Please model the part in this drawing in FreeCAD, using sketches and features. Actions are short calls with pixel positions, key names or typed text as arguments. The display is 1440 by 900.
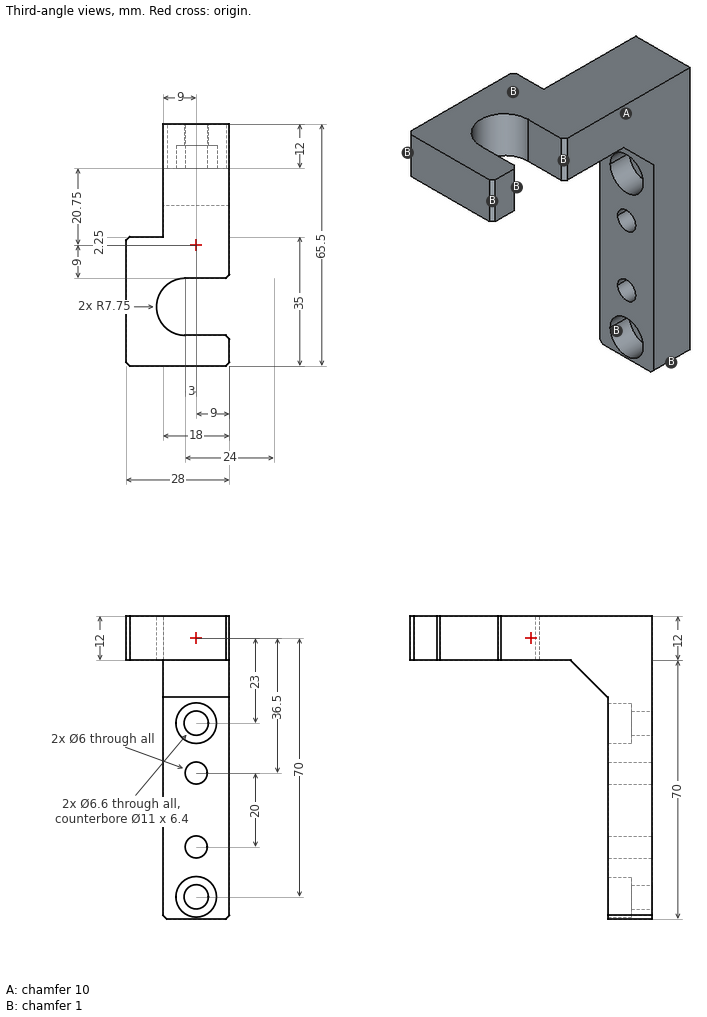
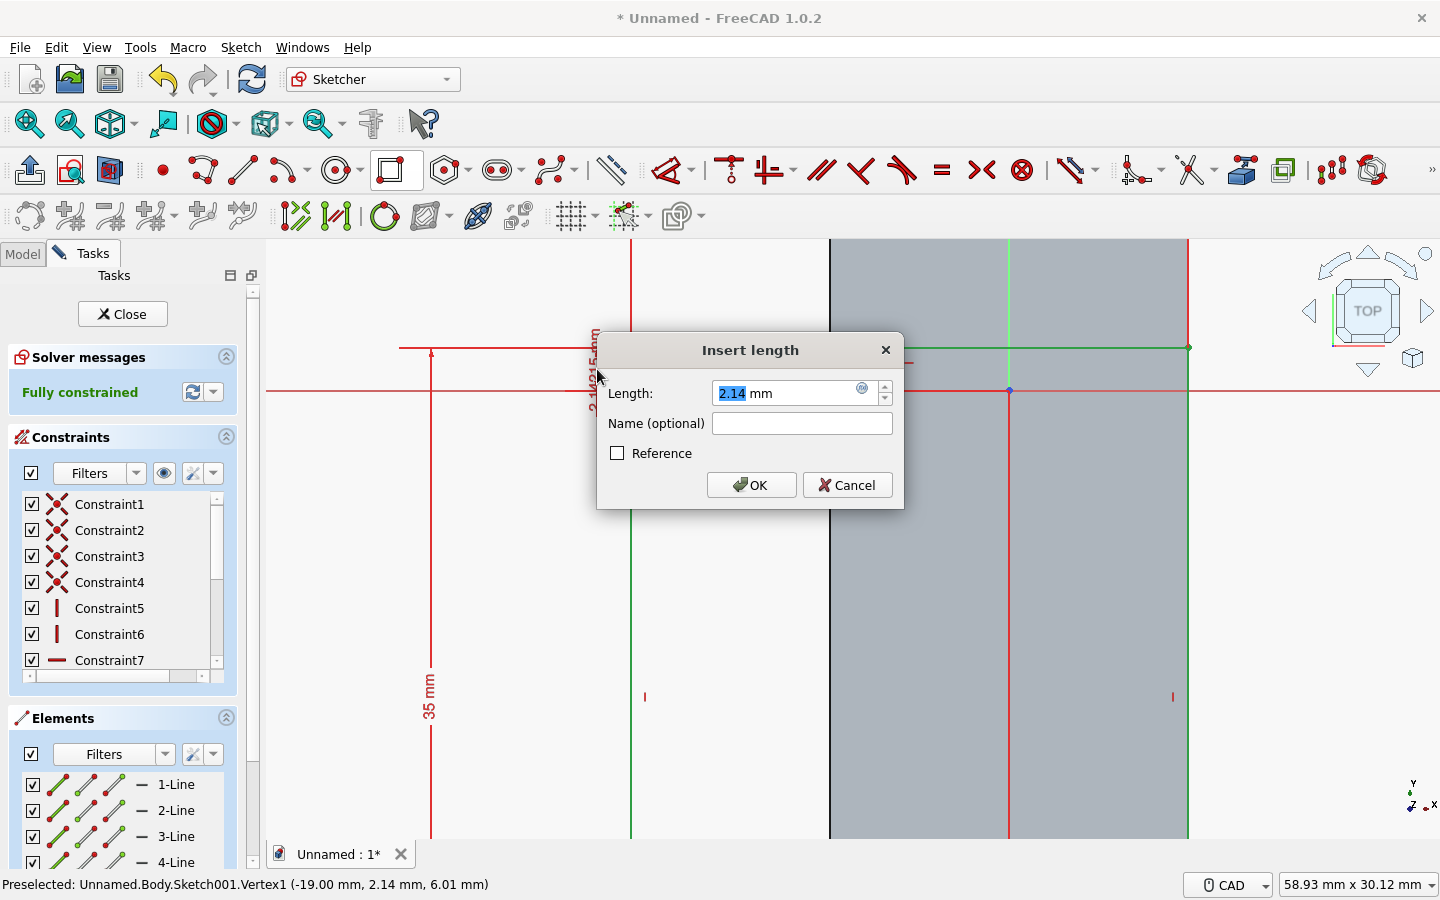
text(2.25)
key(Return)
key(Escape)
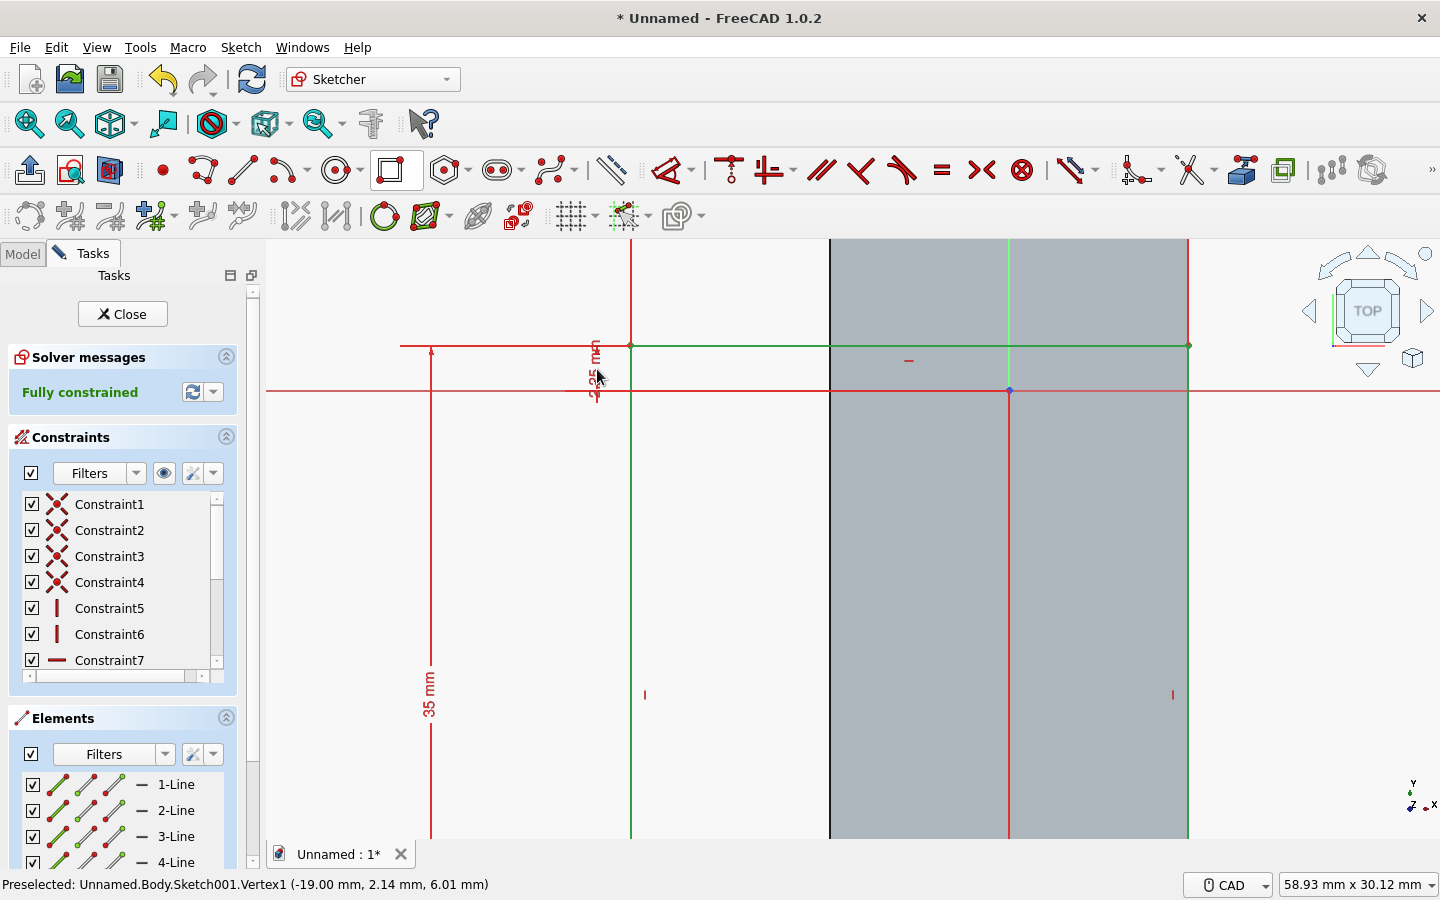
click(123, 314)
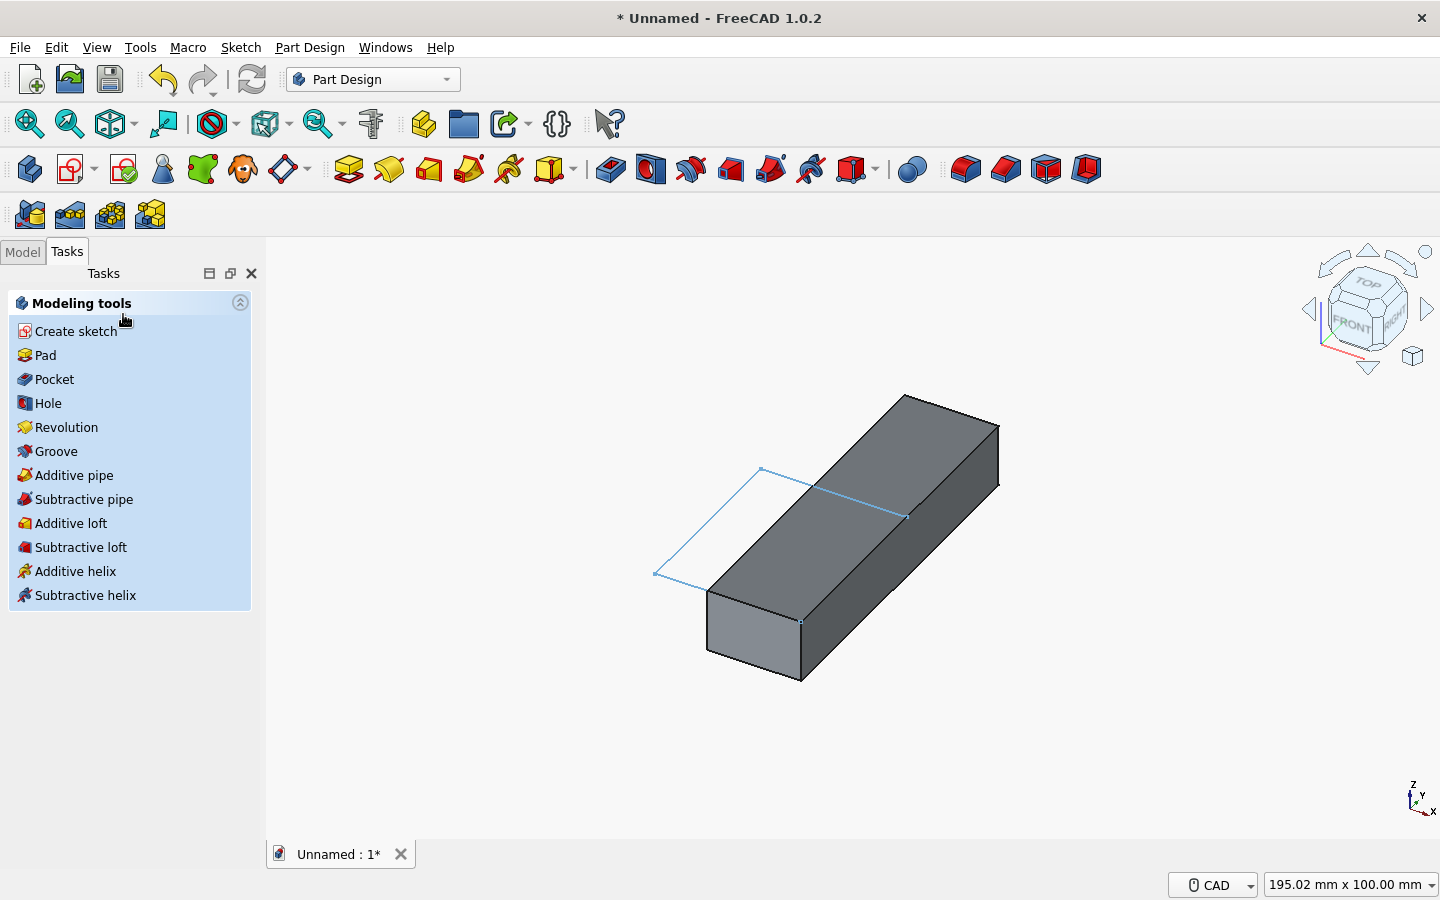
click(350, 170)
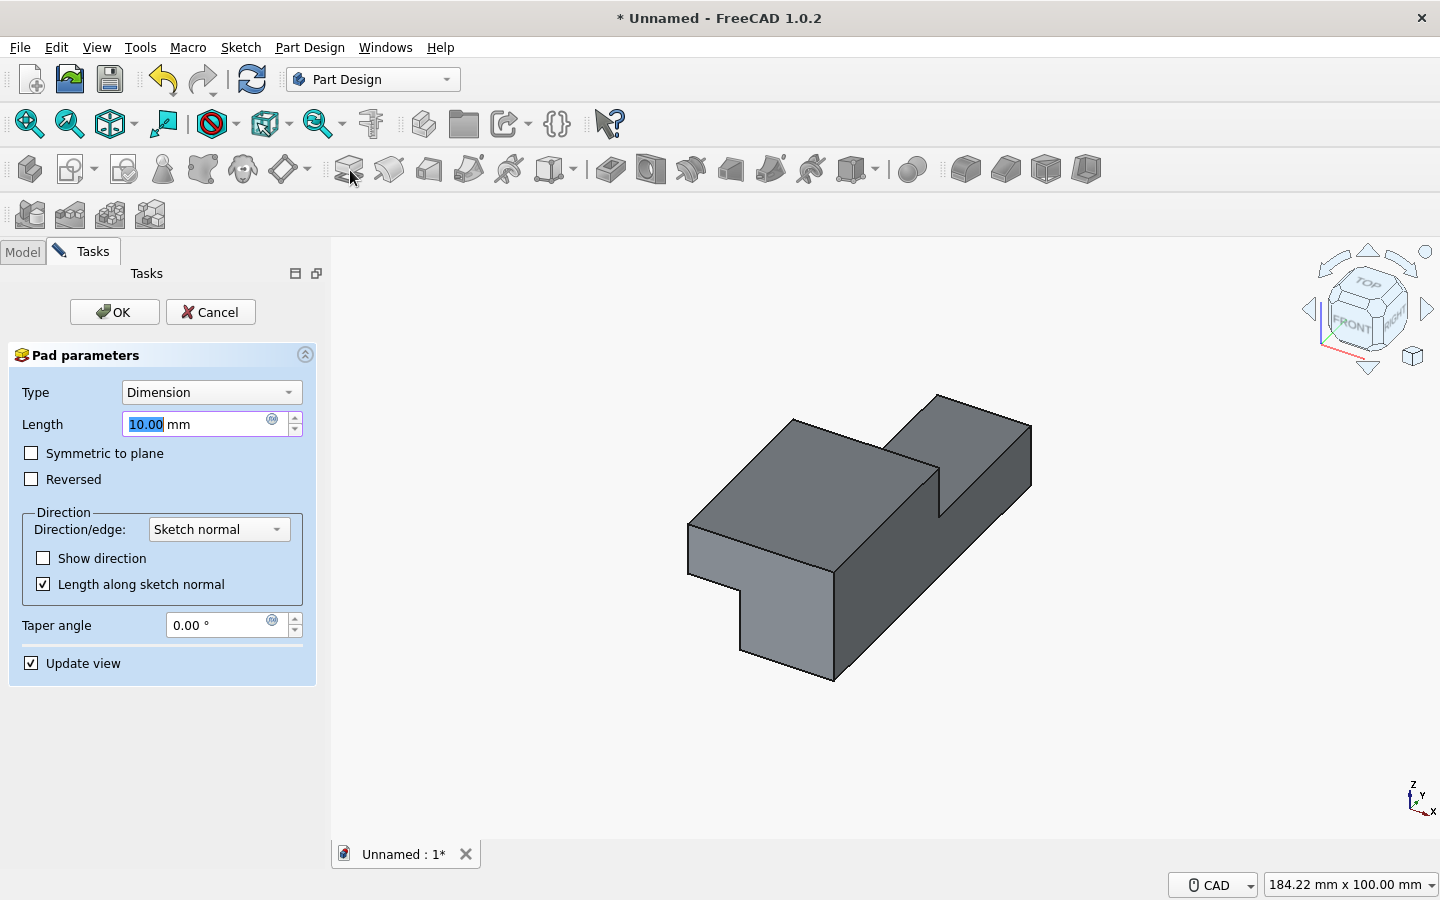
text(12)
key(Tab)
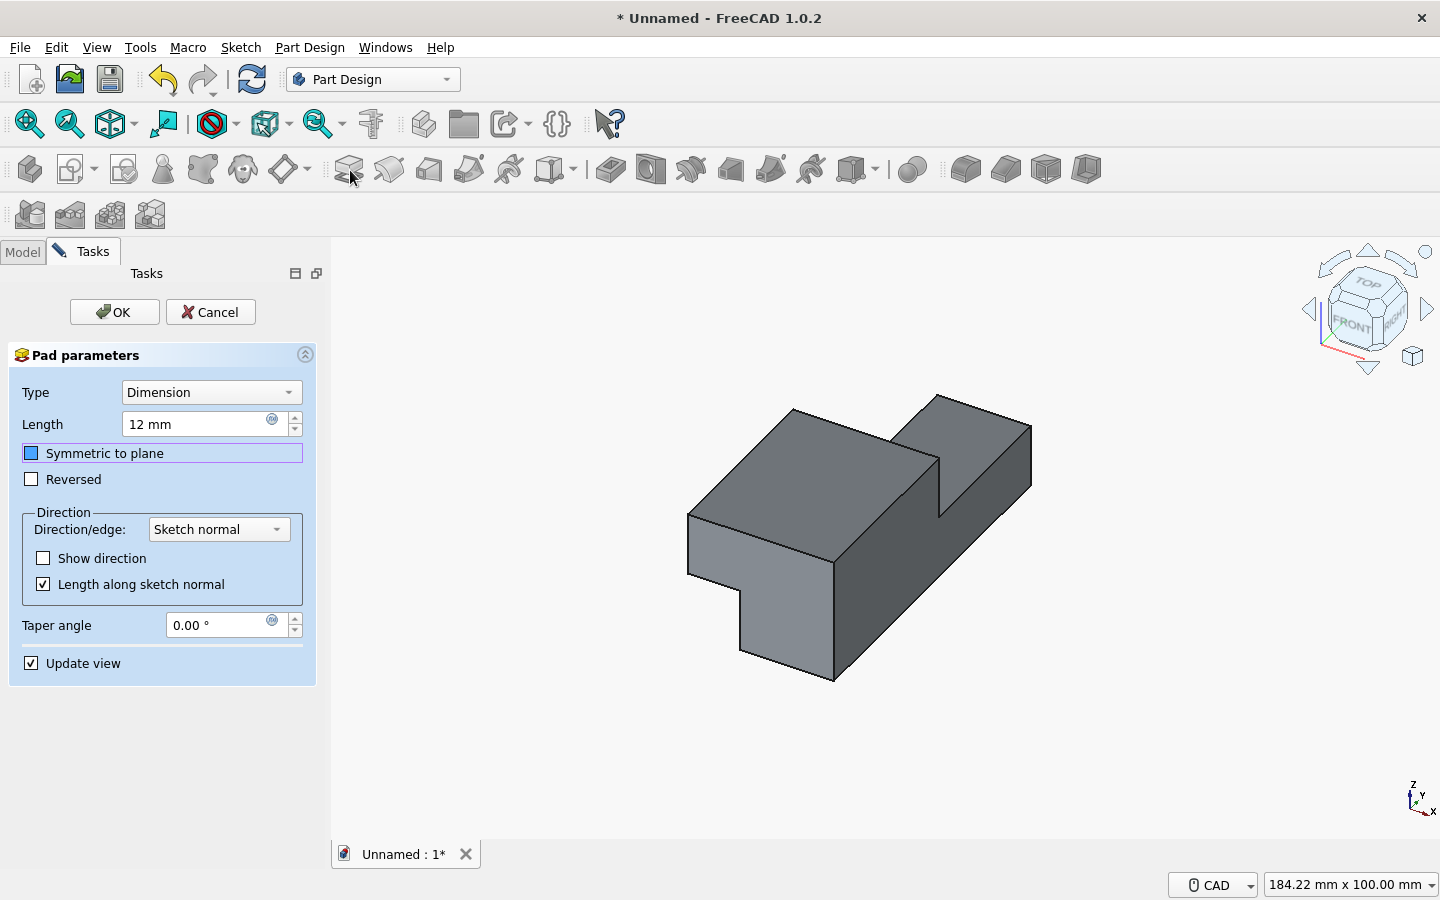
click(30, 479)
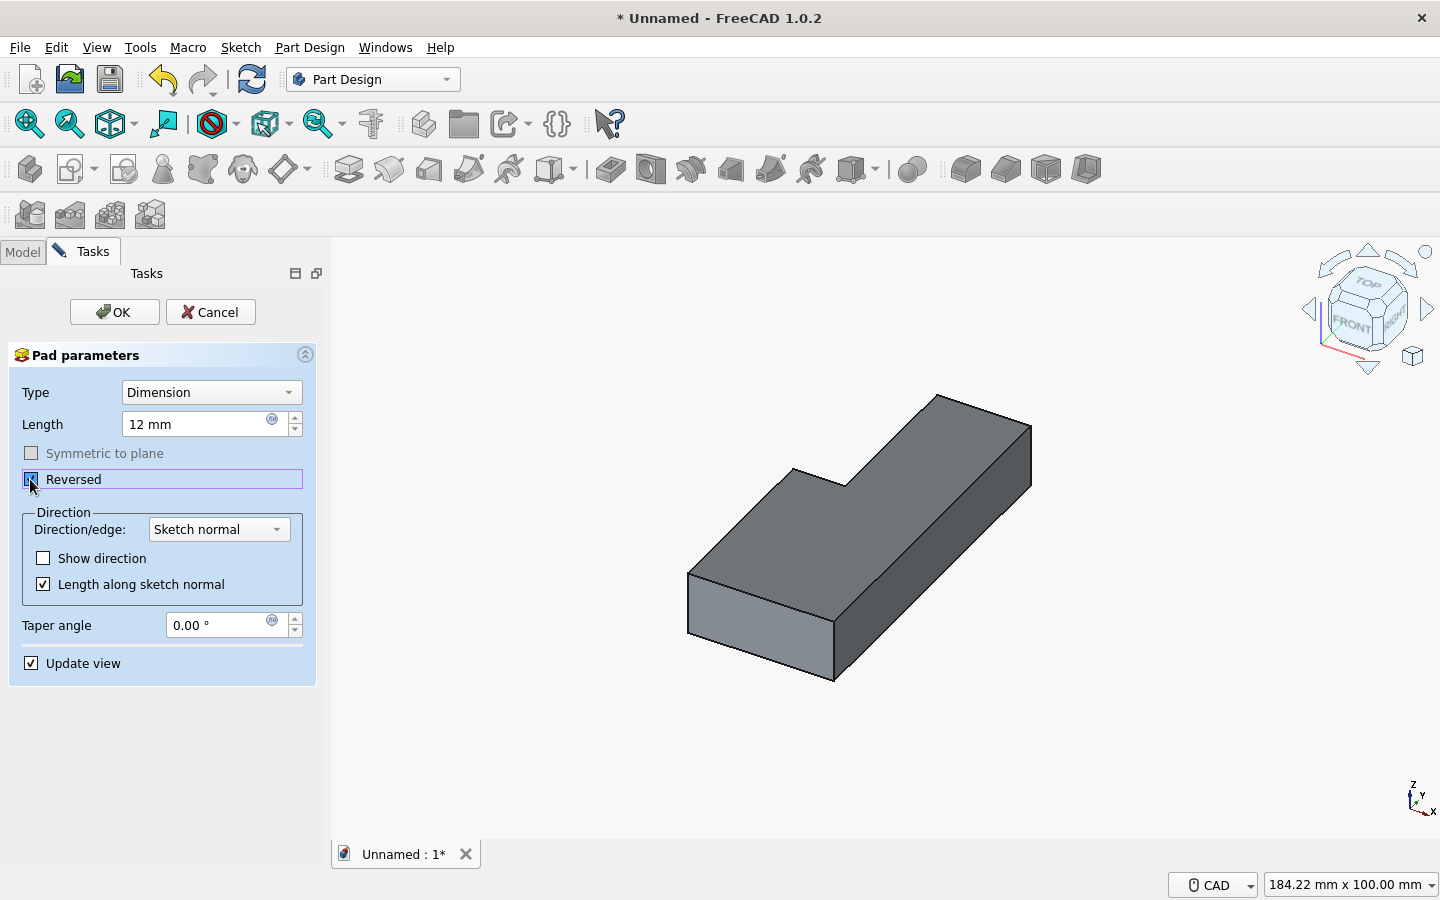
click(115, 312)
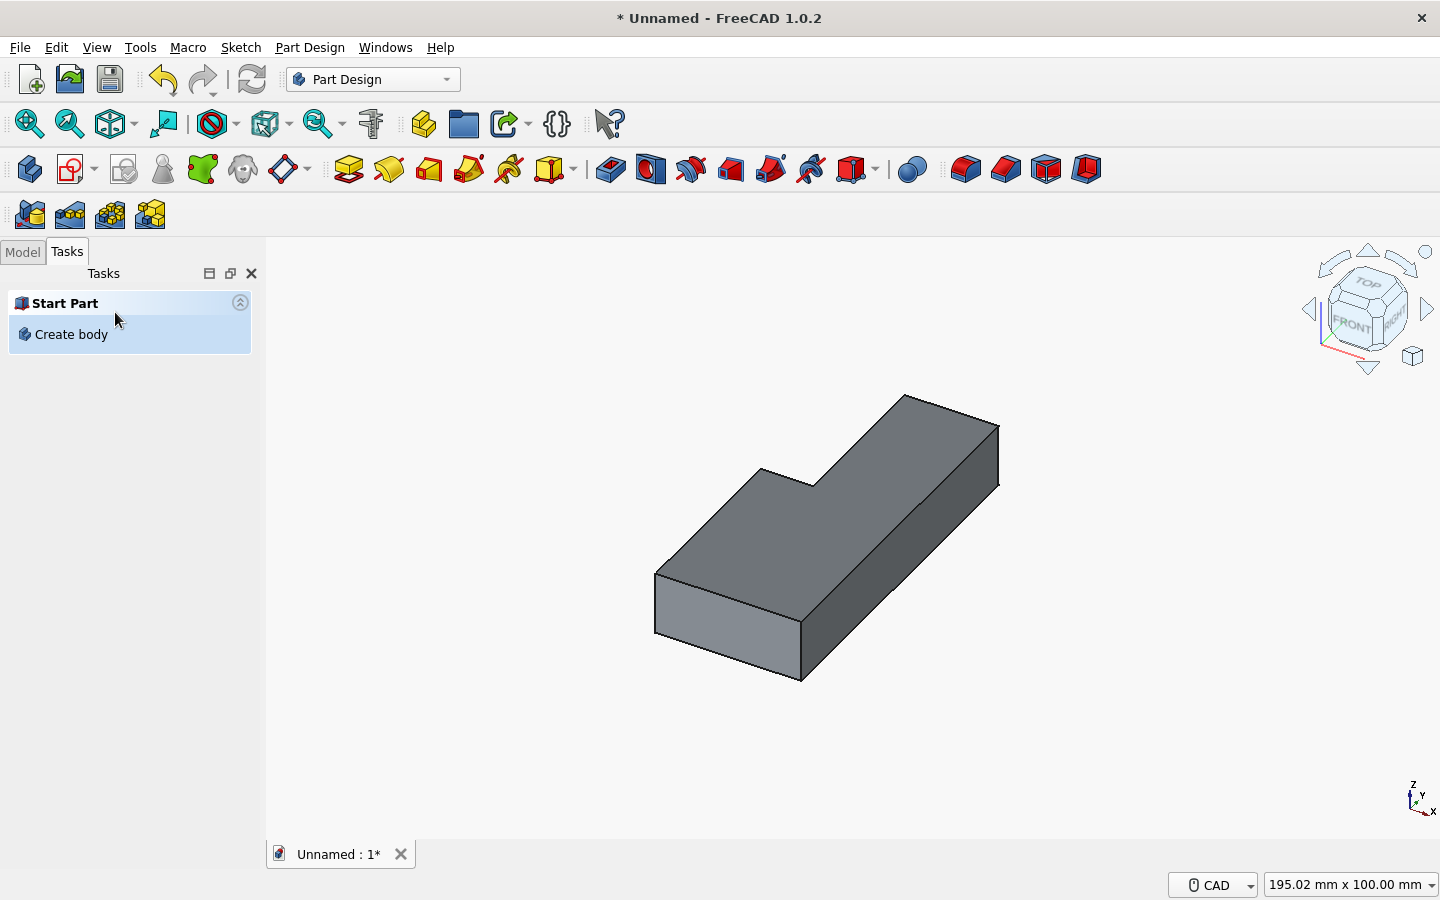
click(771, 555)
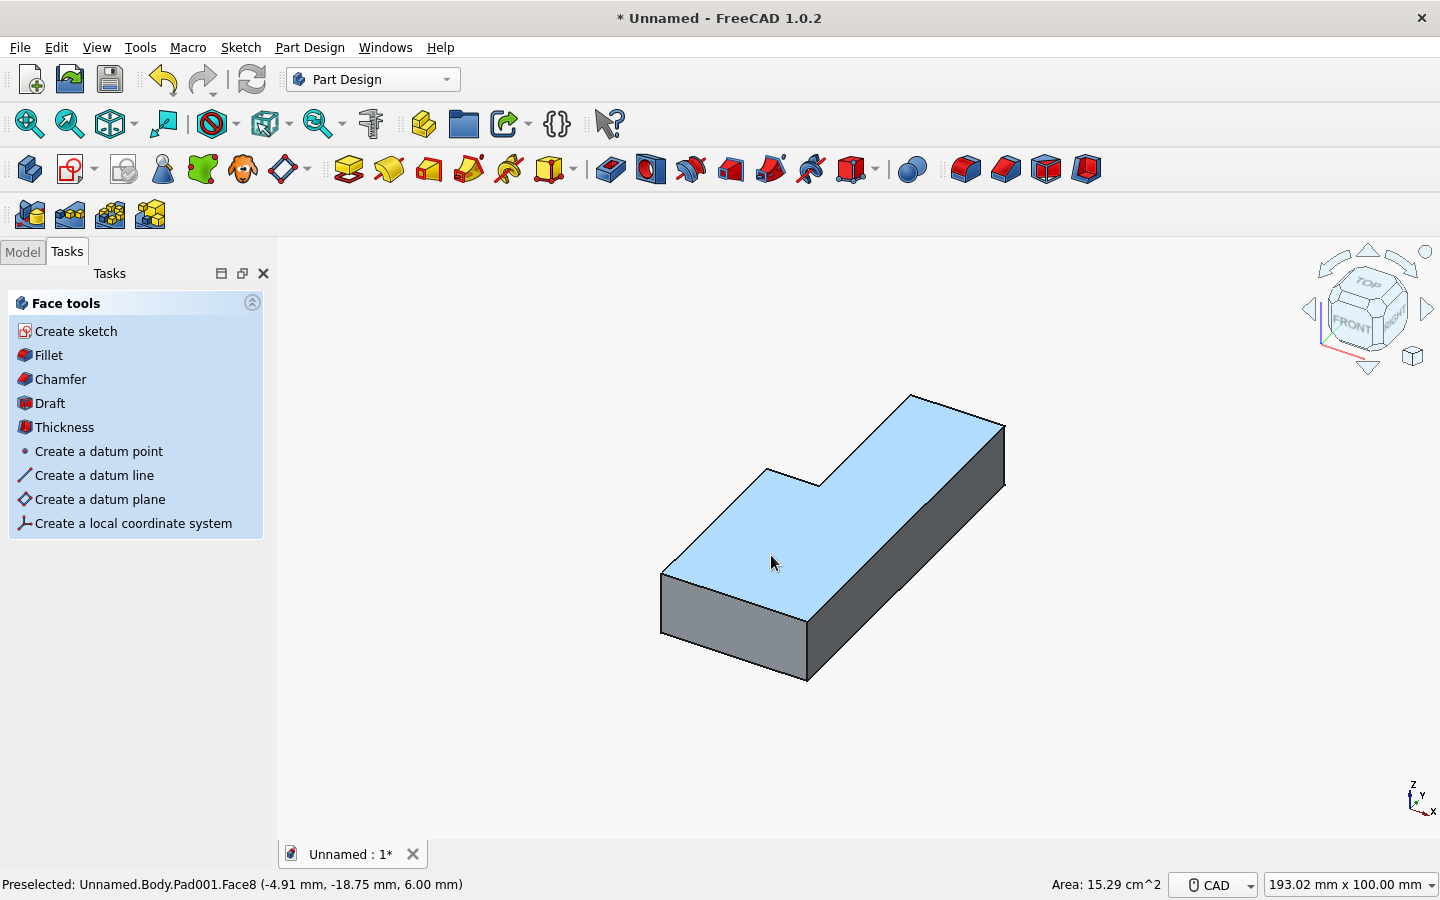
click(70, 170)